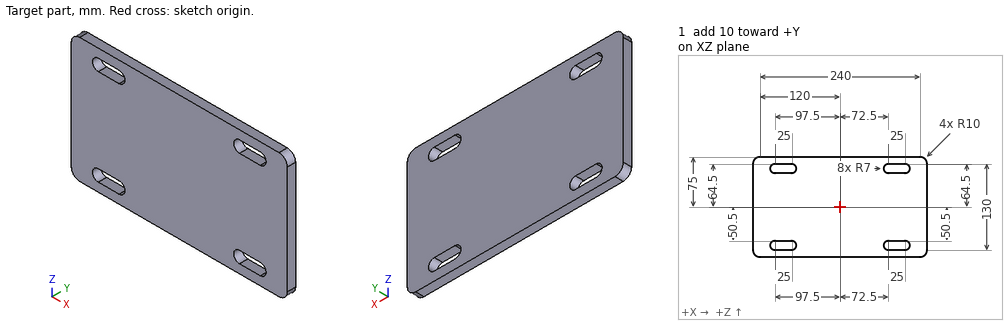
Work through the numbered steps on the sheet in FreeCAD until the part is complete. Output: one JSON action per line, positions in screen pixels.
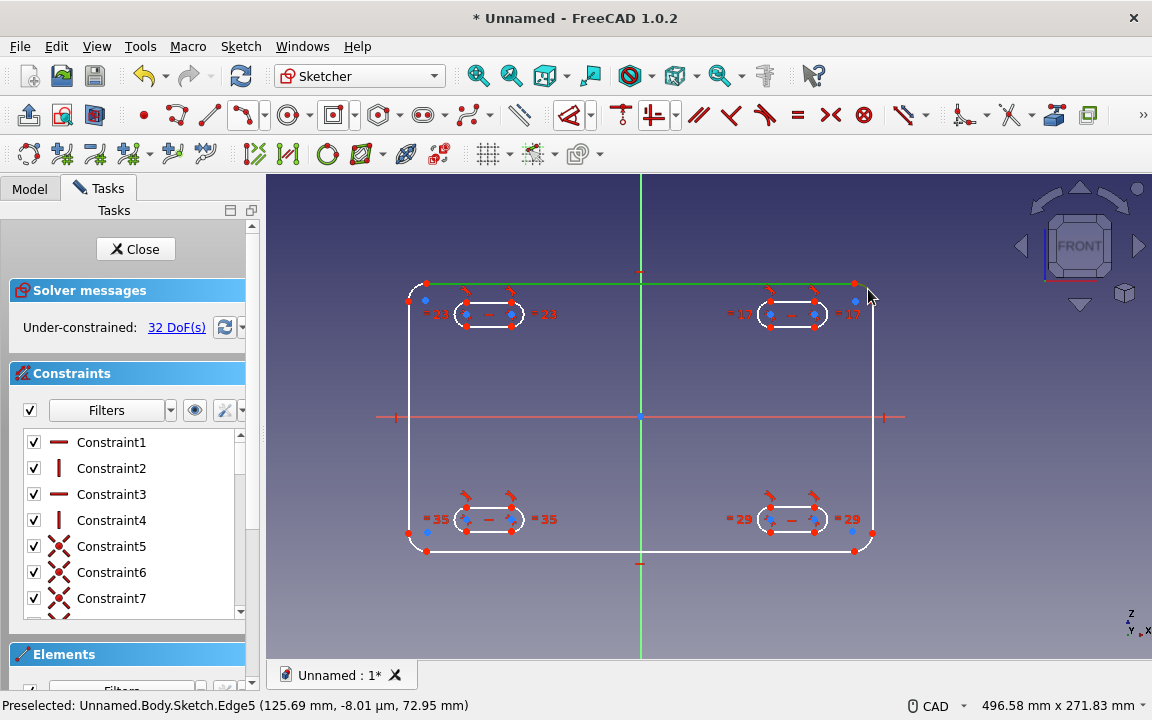
{"action": "left_click", "coordinate": [765, 116]}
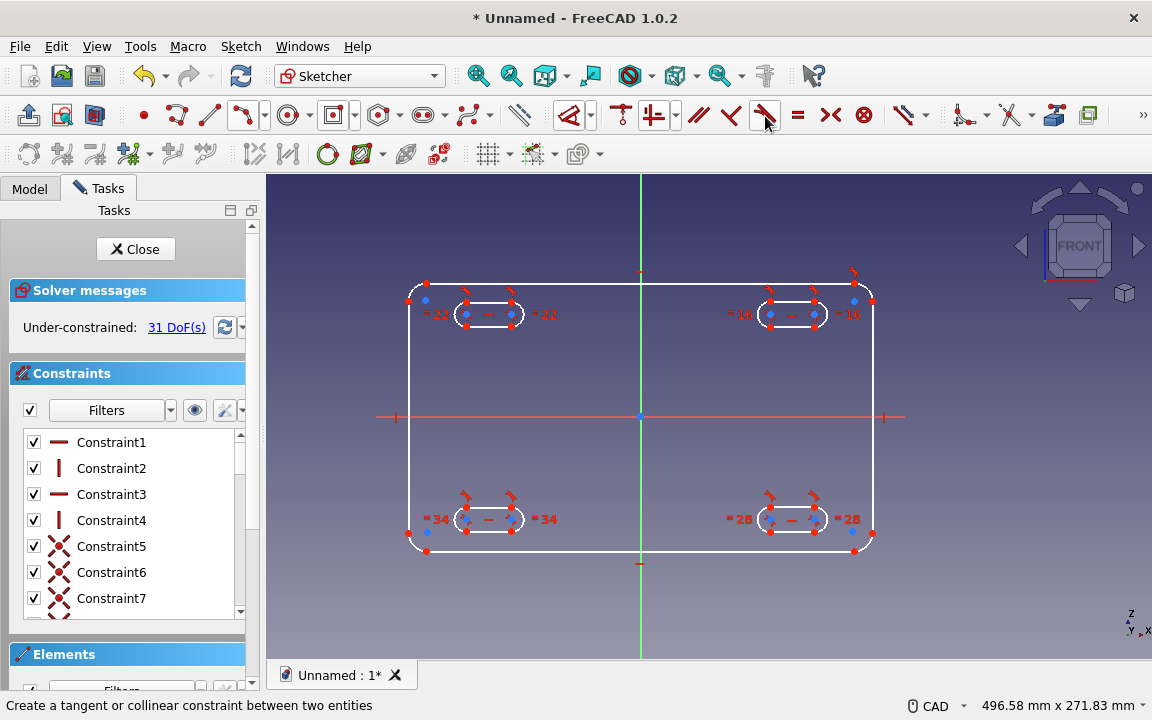
{"action": "left_click", "coordinate": [555, 284]}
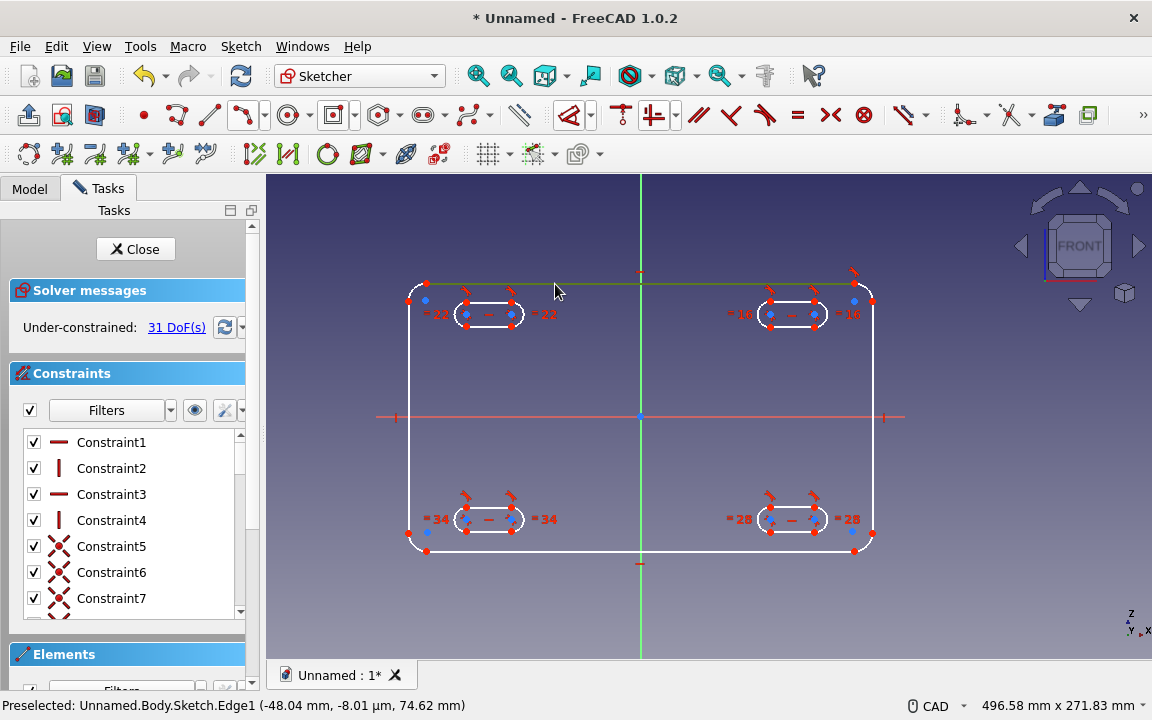
{"action": "left_click", "coordinate": [414, 289]}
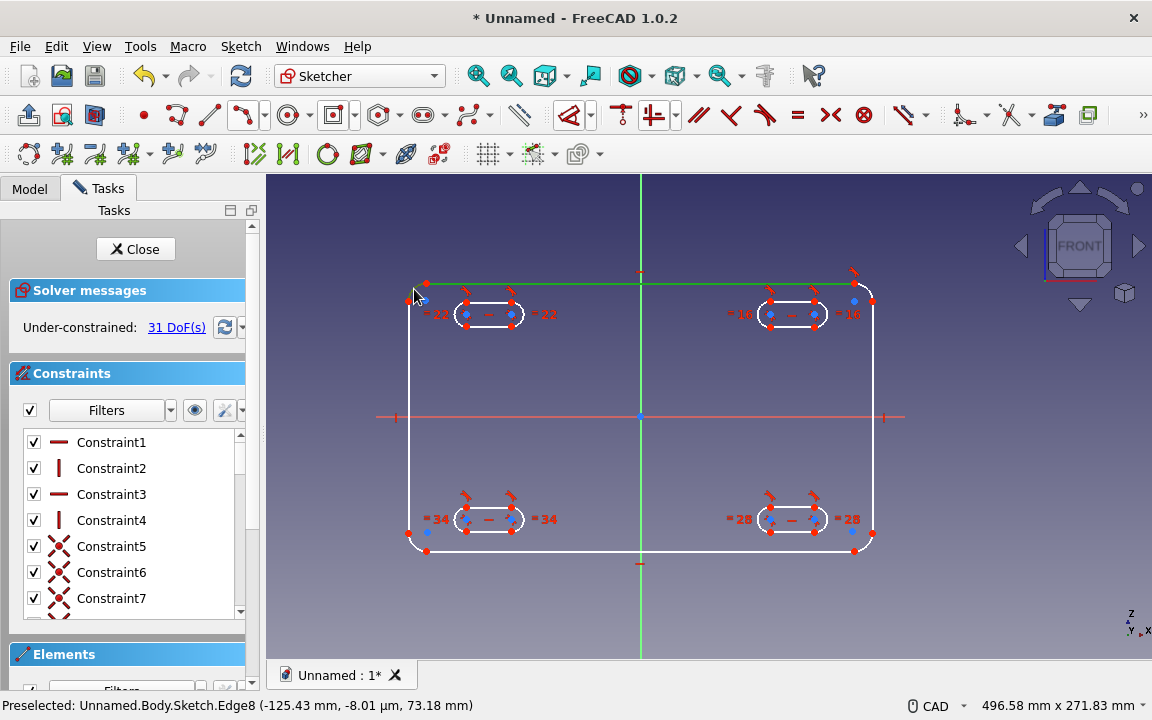
{"action": "left_click", "coordinate": [765, 116]}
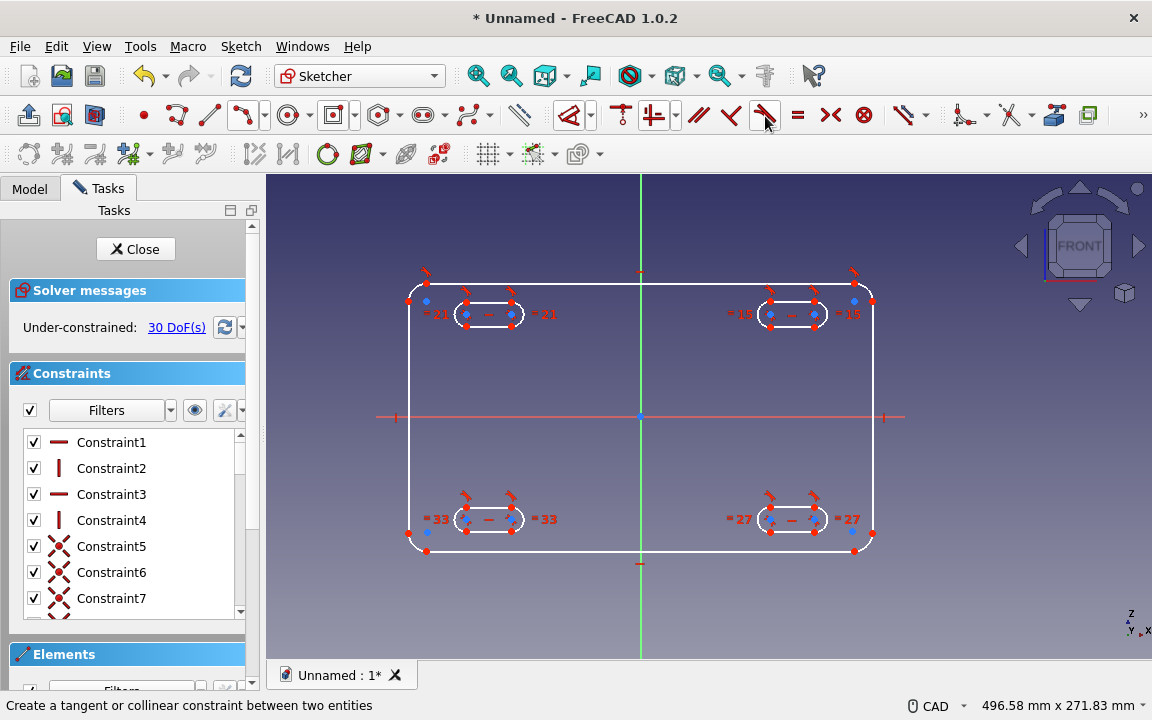
{"action": "left_click", "coordinate": [873, 371]}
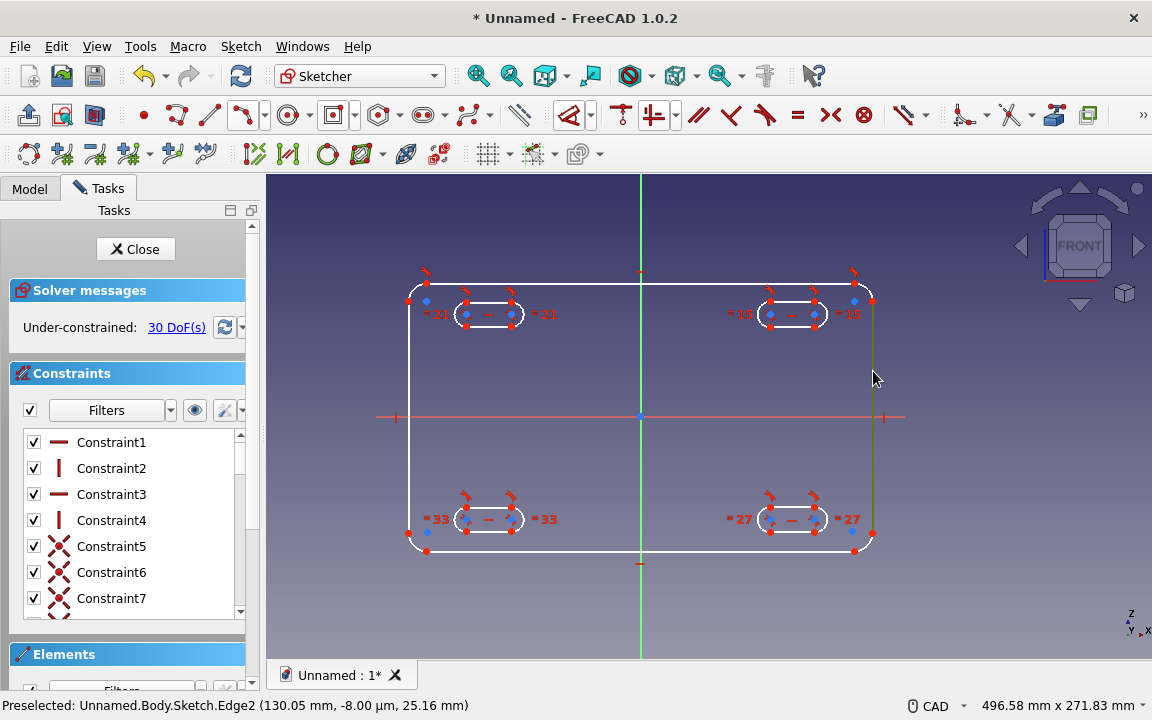
{"action": "left_click", "coordinate": [867, 289]}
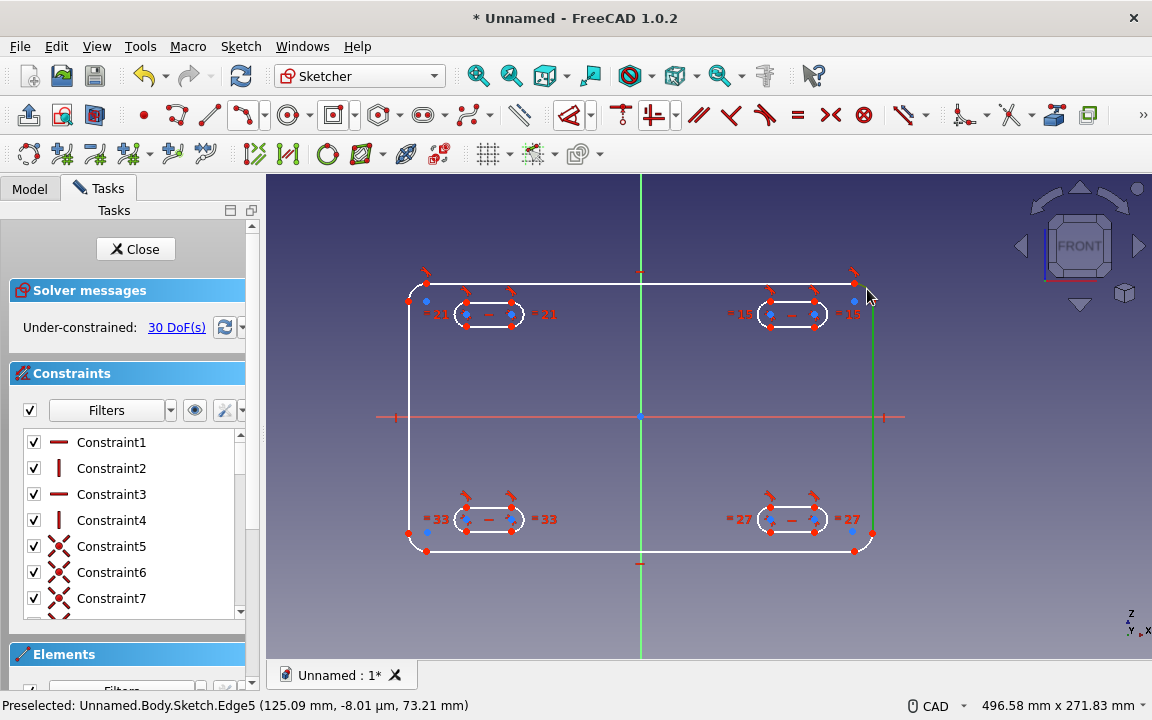
{"action": "left_click", "coordinate": [765, 116]}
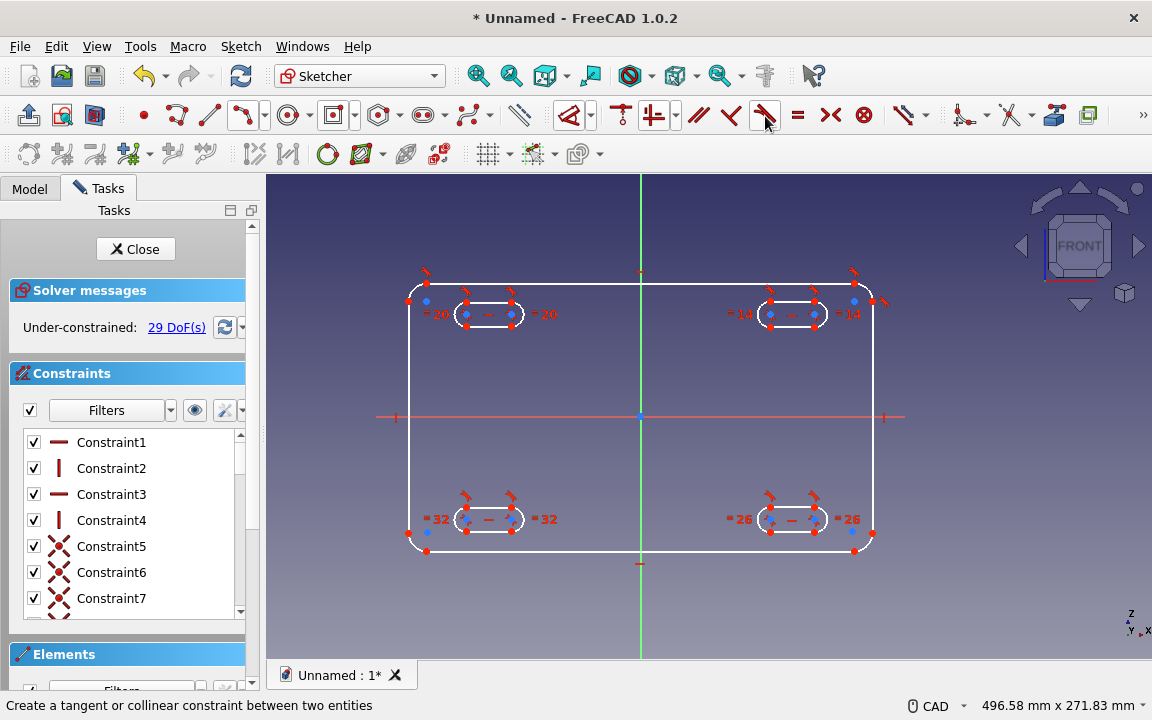
{"action": "left_click", "coordinate": [873, 371]}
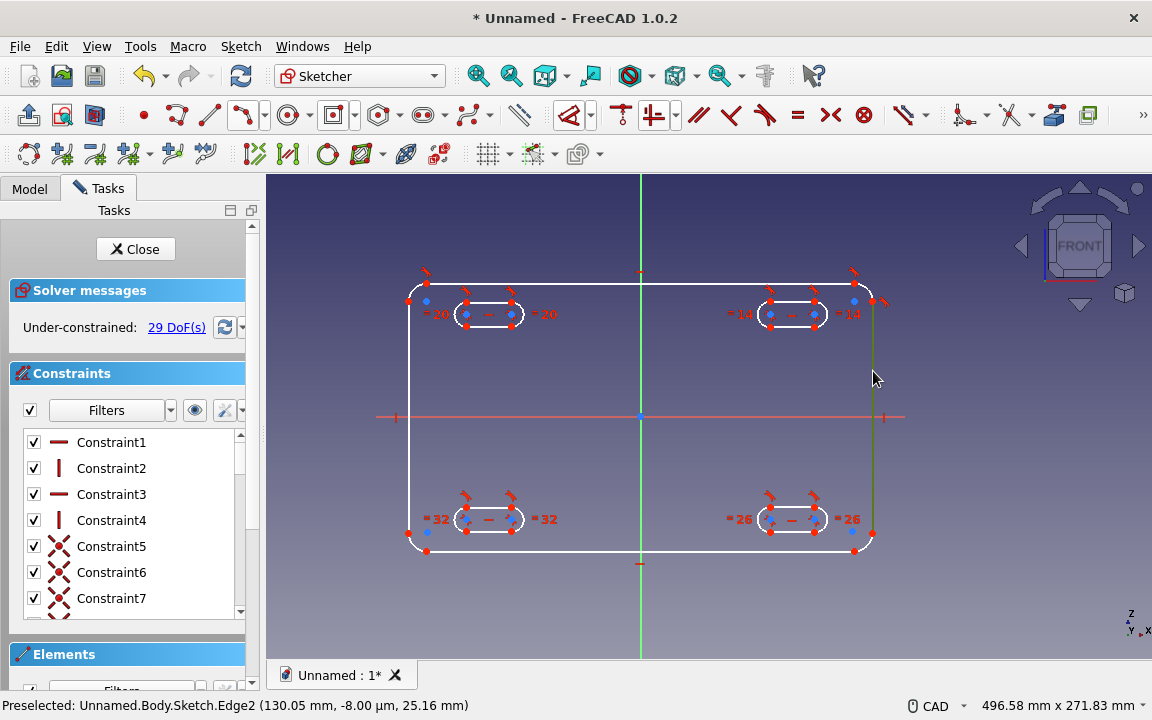
{"action": "left_click", "coordinate": [867, 546]}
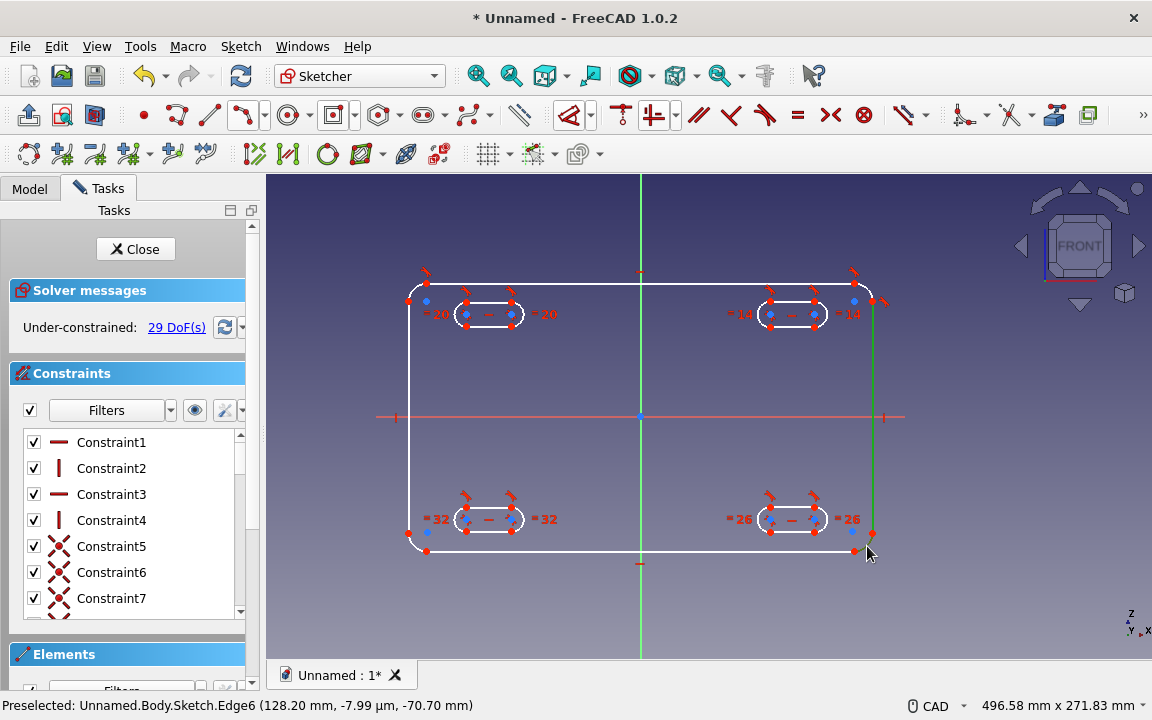
{"action": "left_click", "coordinate": [765, 116]}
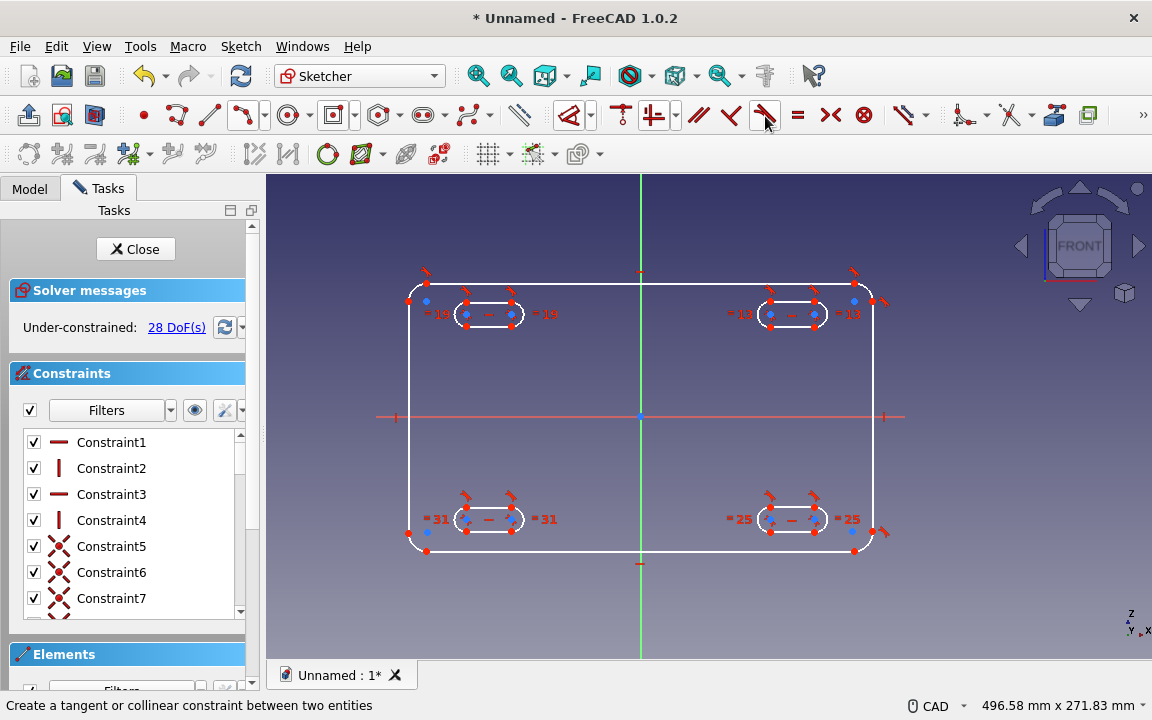
{"action": "left_click", "coordinate": [726, 552]}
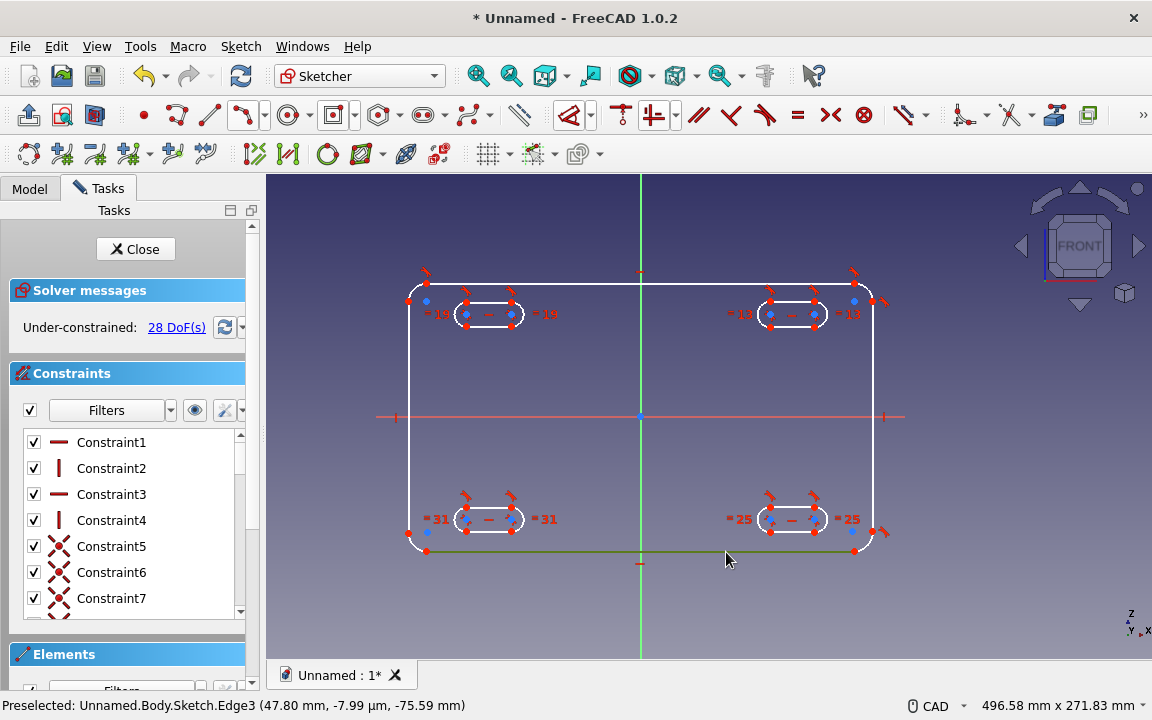
{"action": "left_click", "coordinate": [868, 545]}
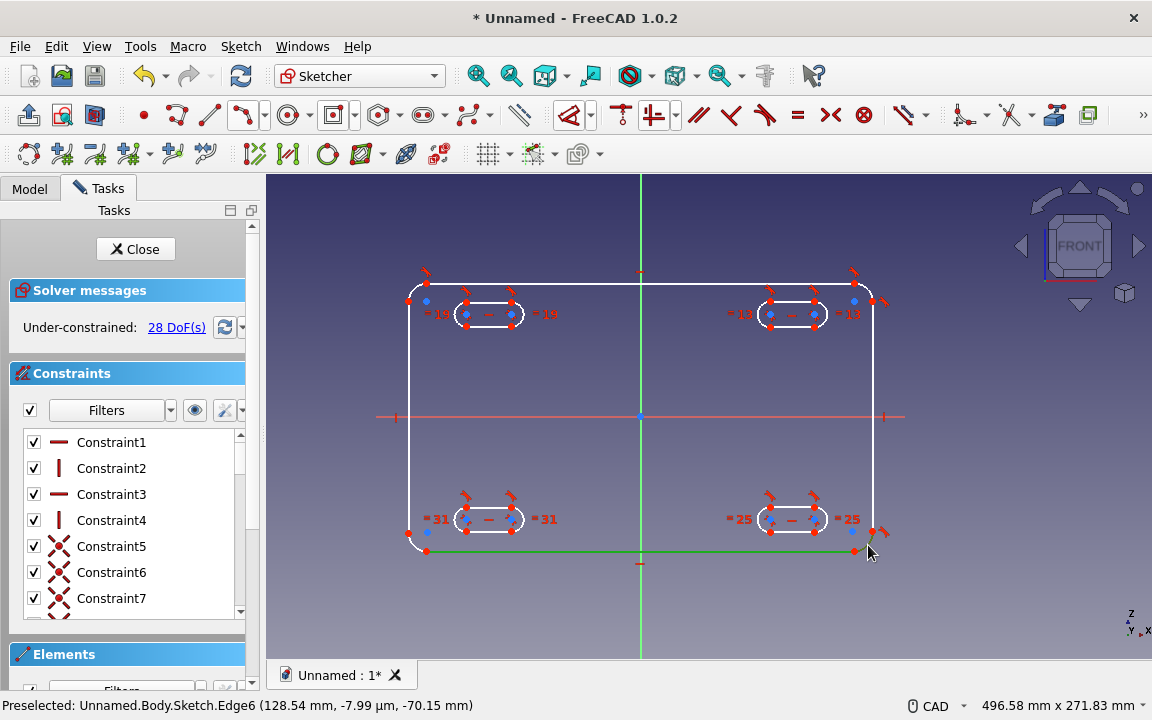
{"action": "left_click", "coordinate": [765, 116]}